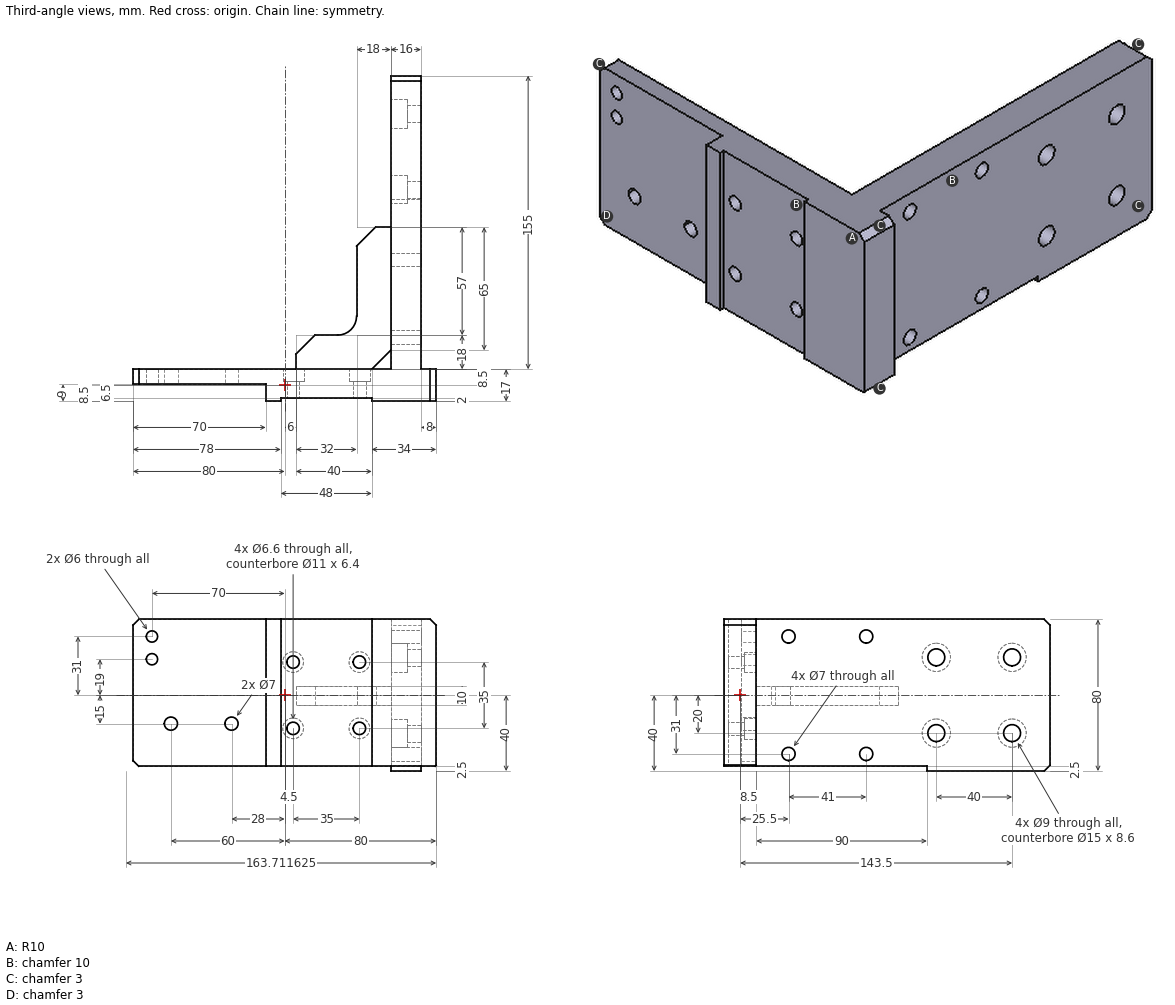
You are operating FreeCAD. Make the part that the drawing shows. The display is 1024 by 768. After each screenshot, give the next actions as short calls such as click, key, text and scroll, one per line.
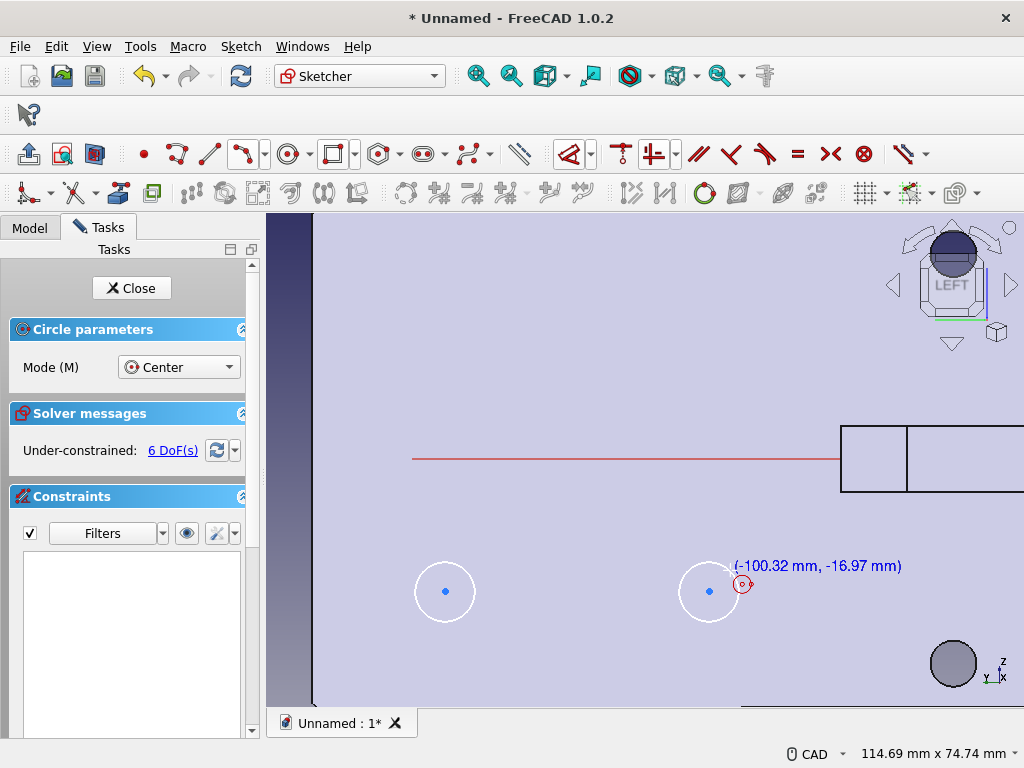
click(709, 327)
click(730, 306)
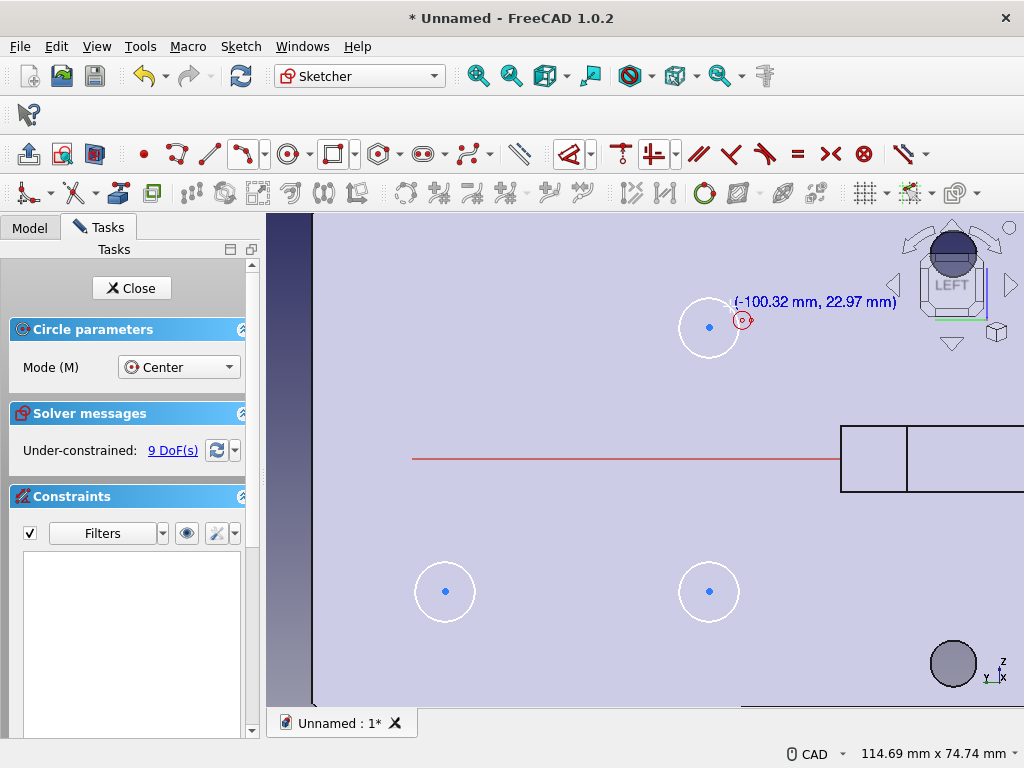
click(445, 327)
click(466, 306)
key(Escape)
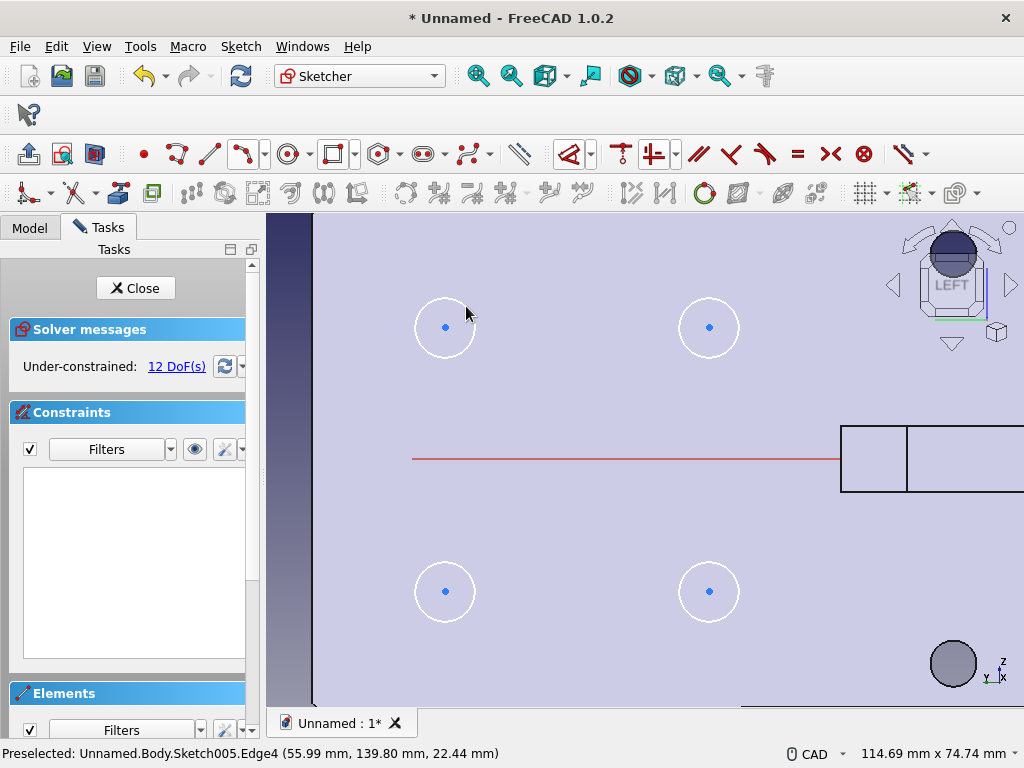
click(466, 571)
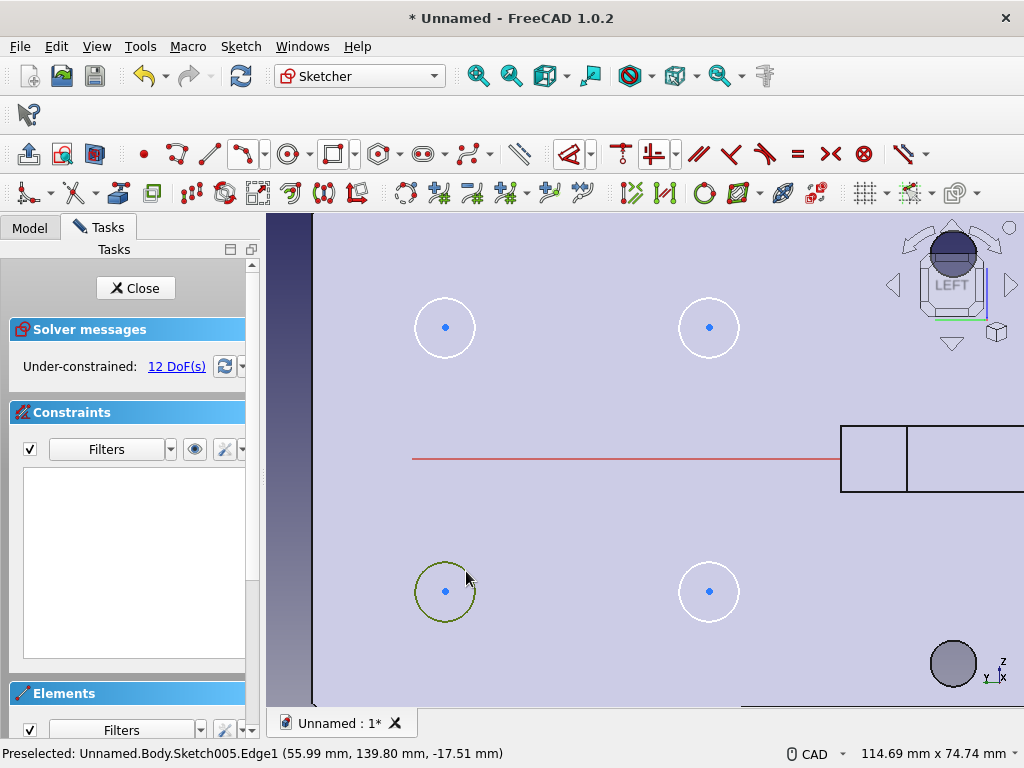
click(730, 571)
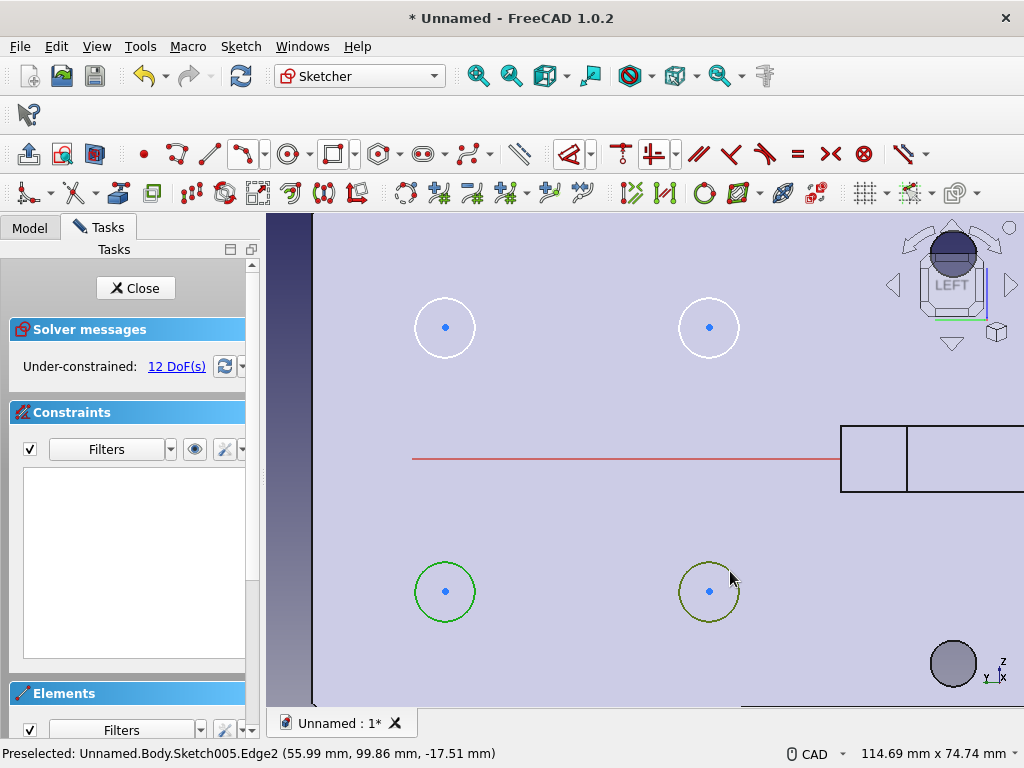
click(730, 307)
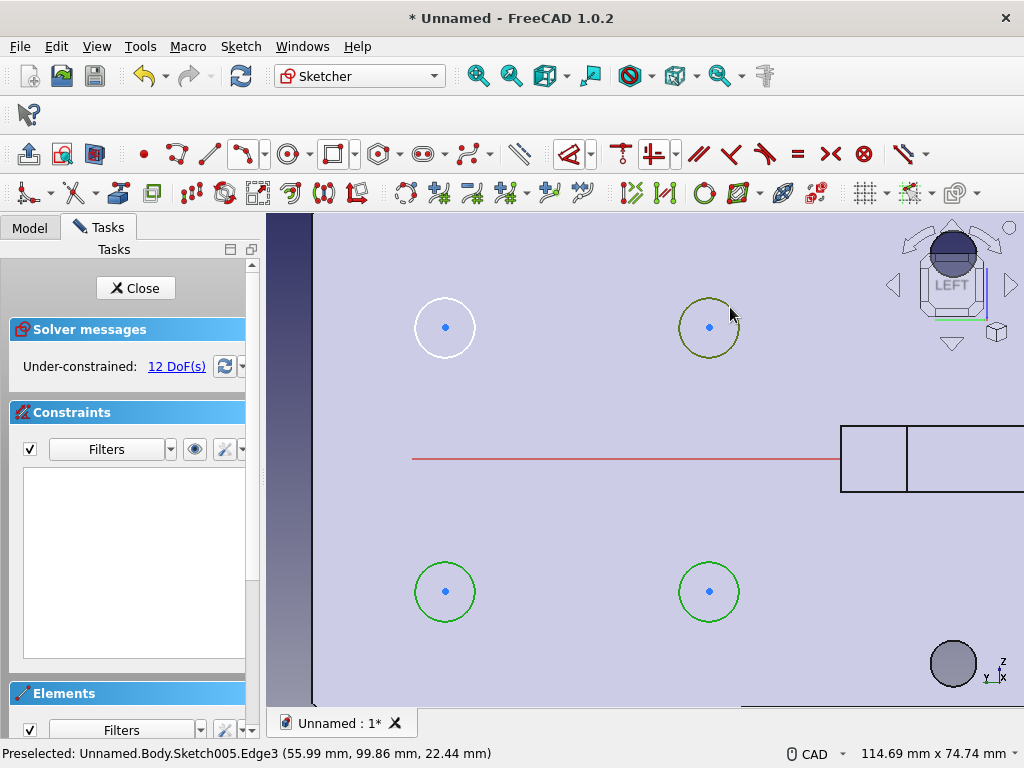
click(466, 307)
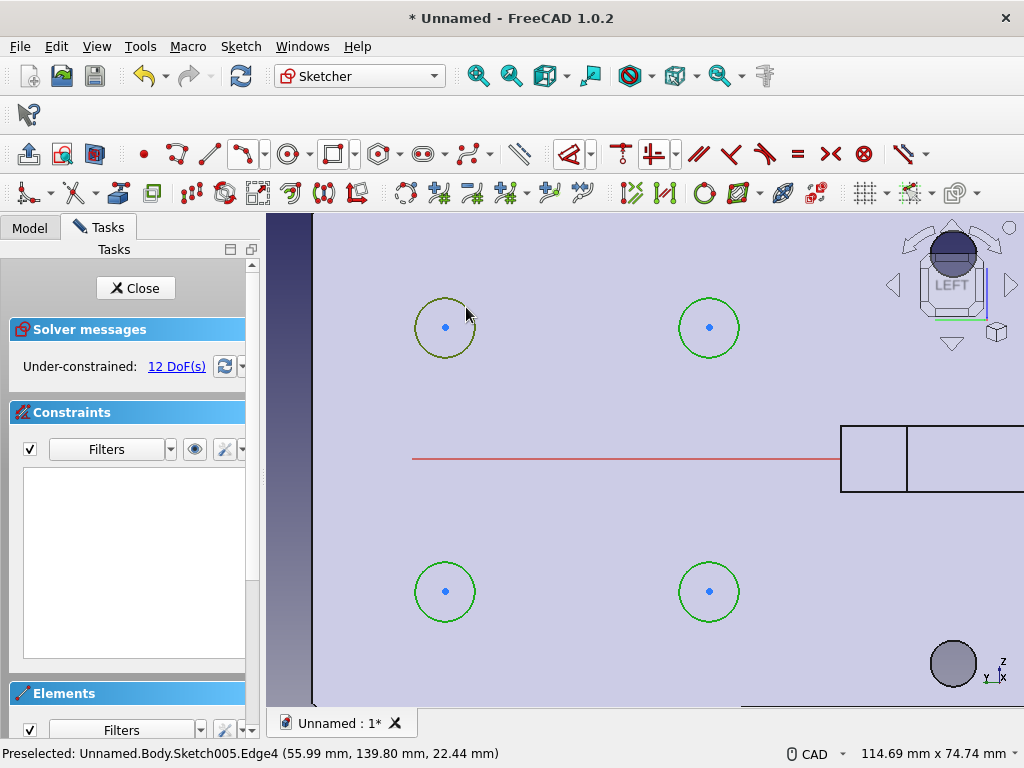
click(798, 154)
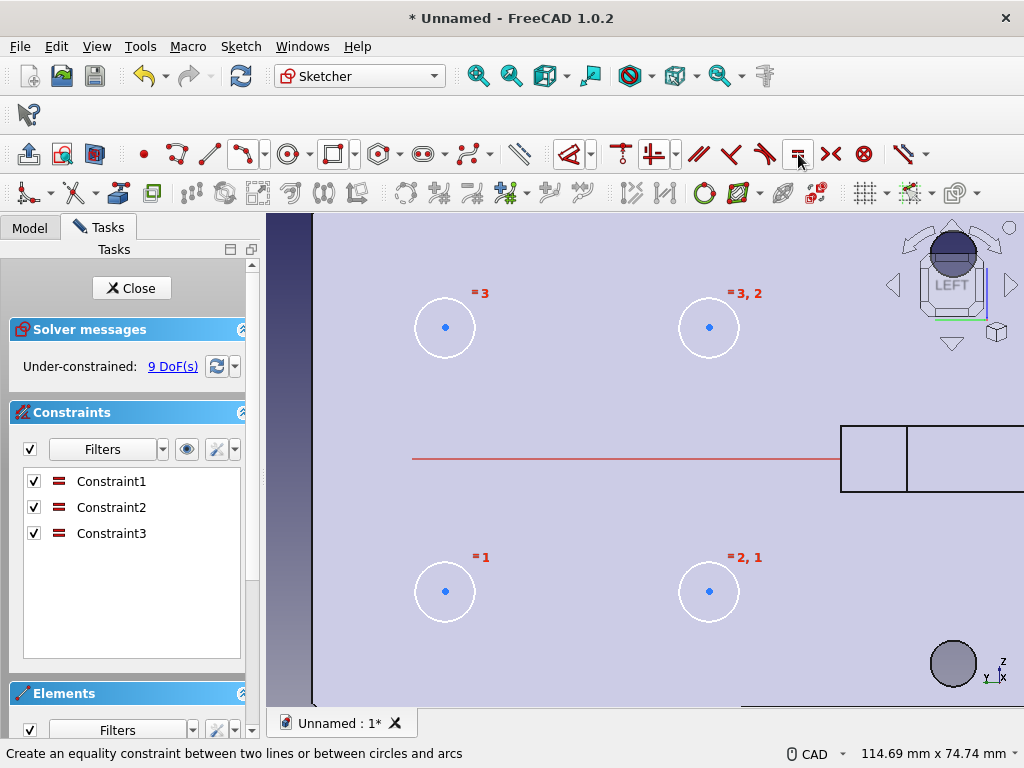
click(709, 592)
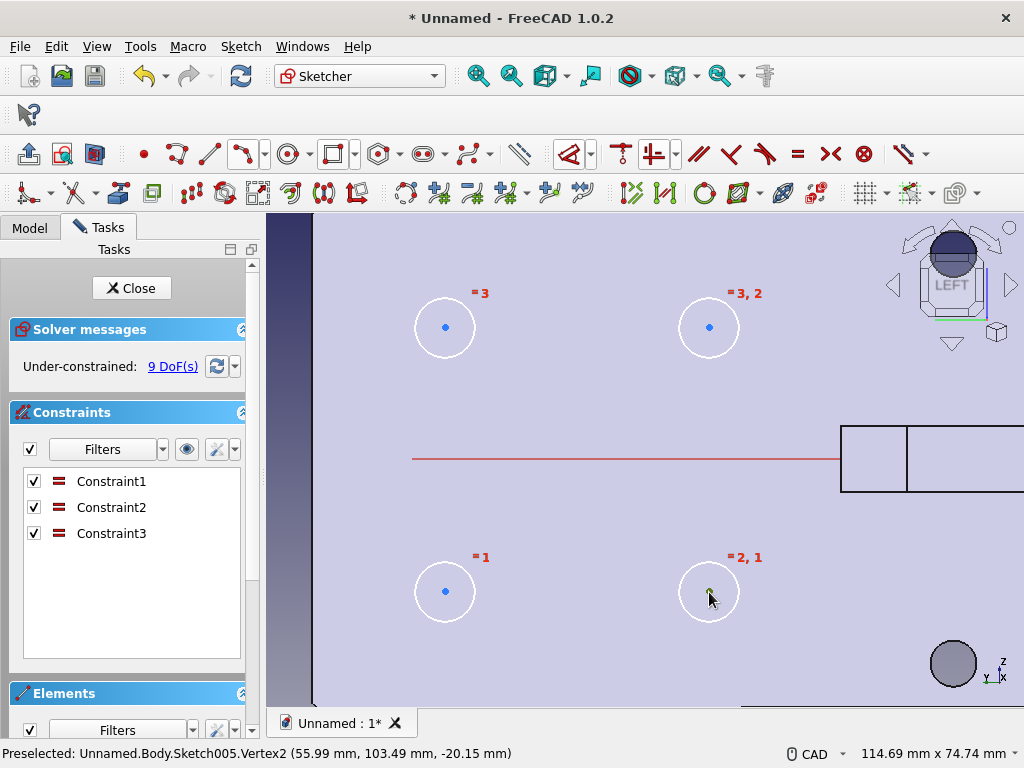
click(709, 328)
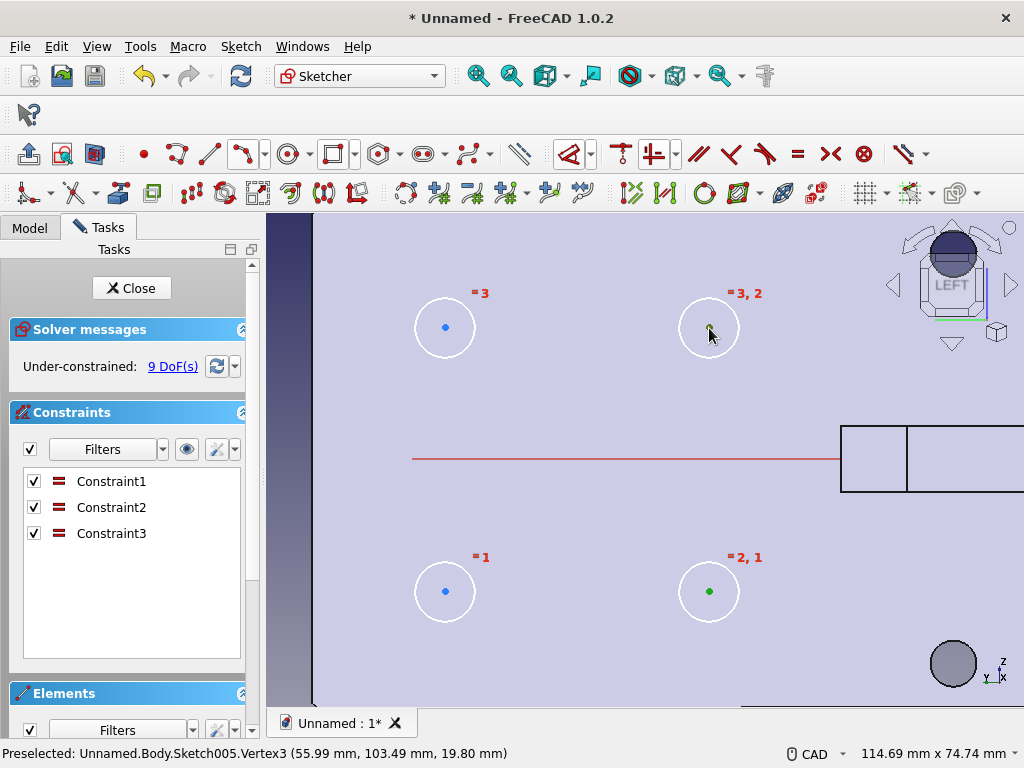
click(415, 459)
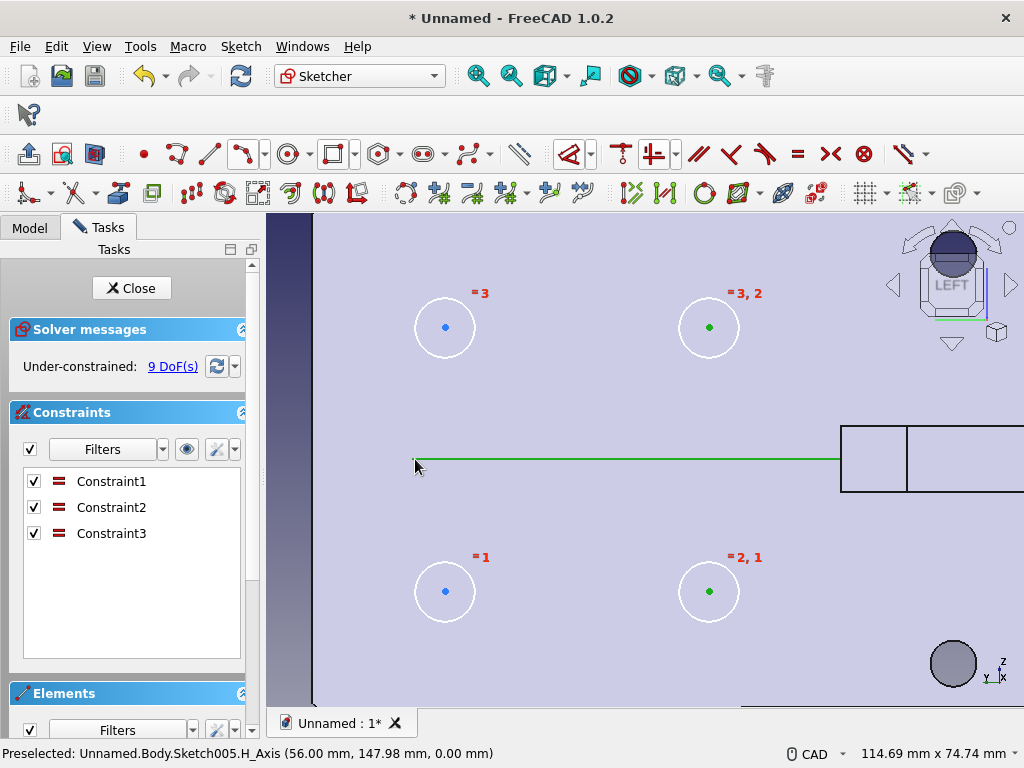
click(831, 154)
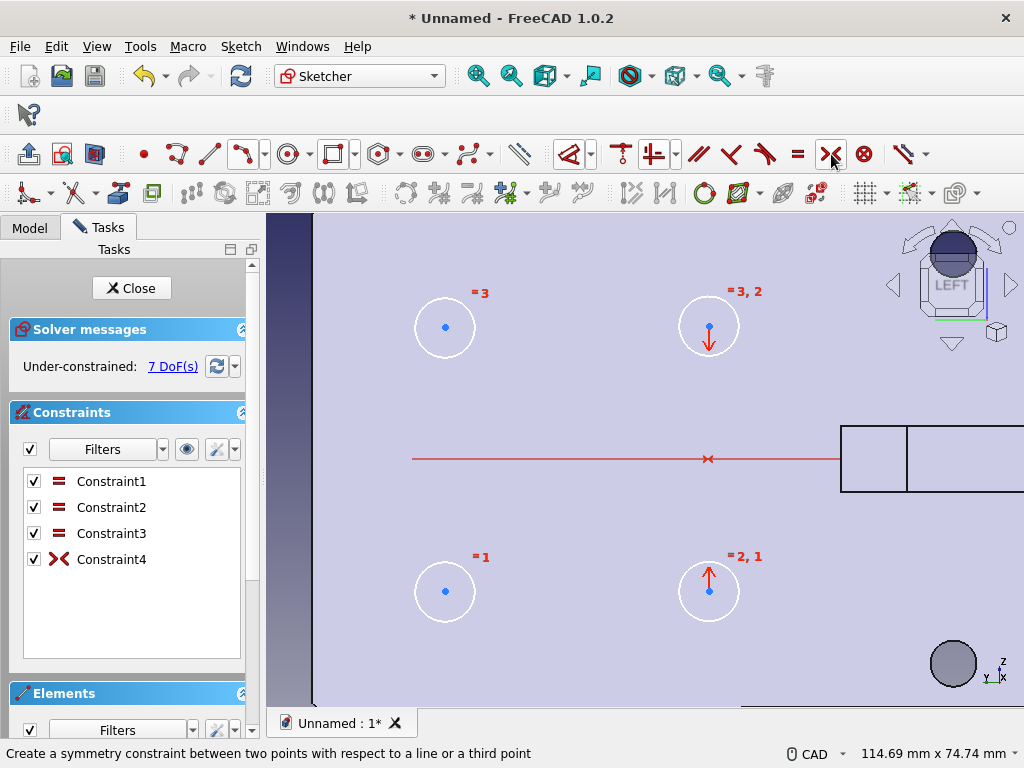
click(445, 592)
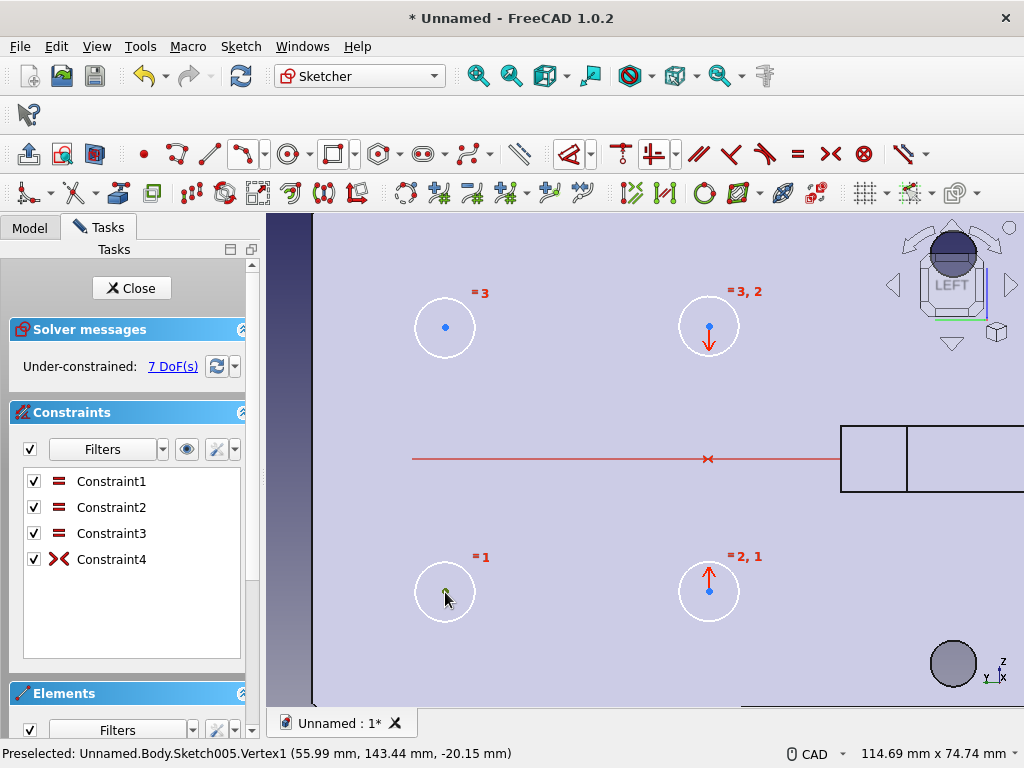
click(445, 328)